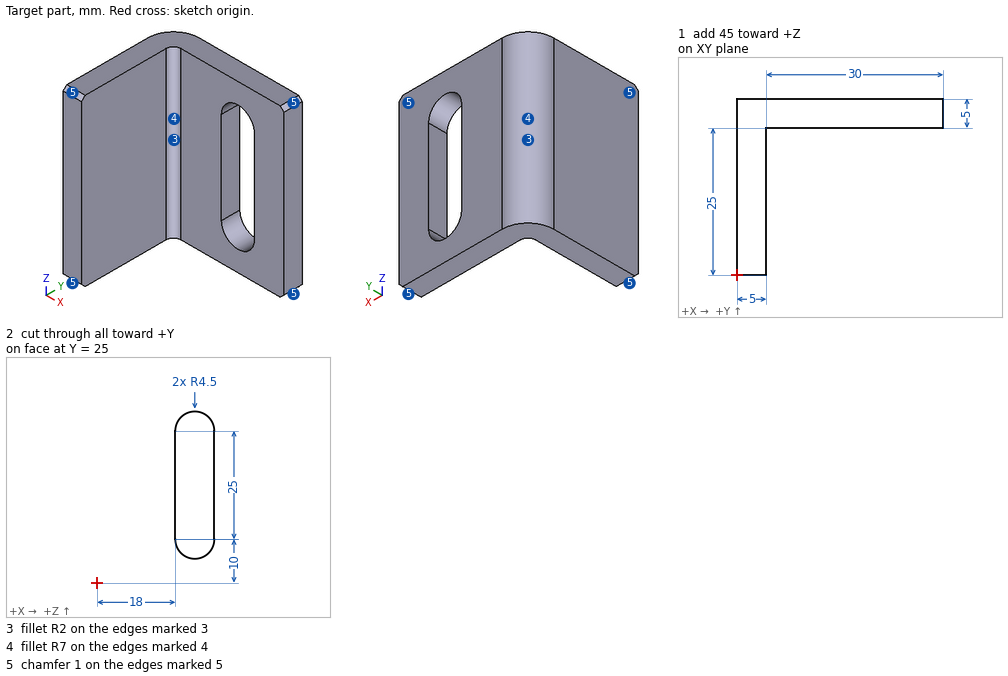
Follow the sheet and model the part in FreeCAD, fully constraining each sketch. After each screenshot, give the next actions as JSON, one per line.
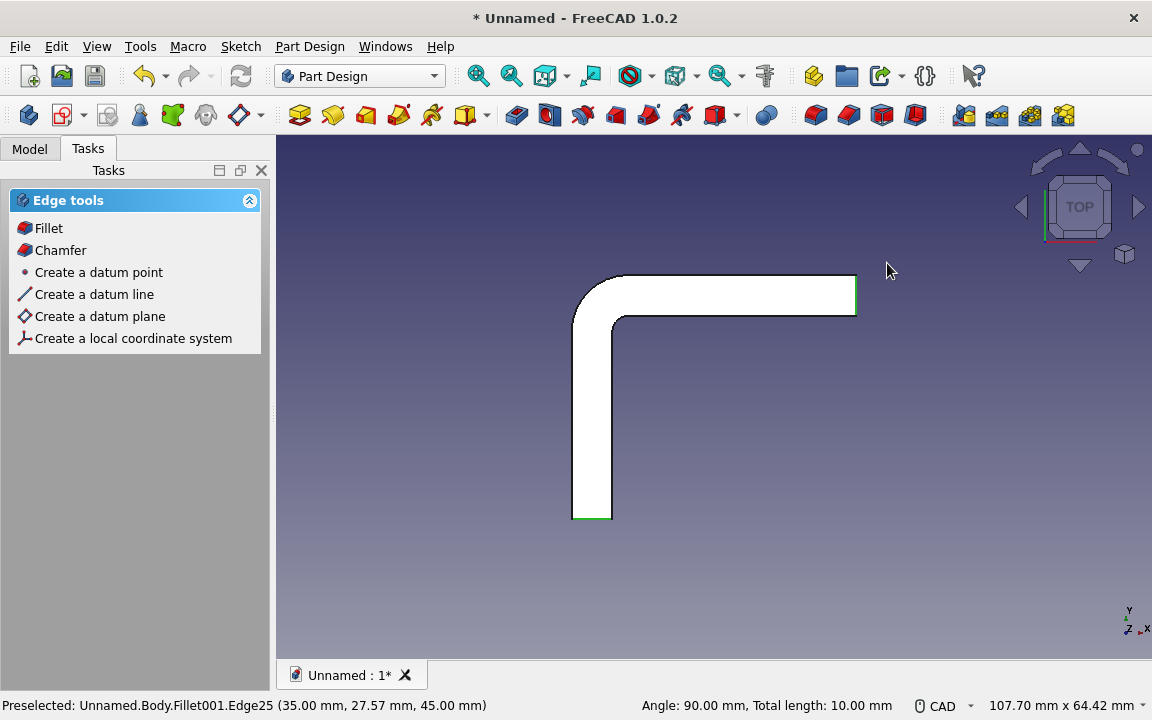
{"action": "key", "text": "1"}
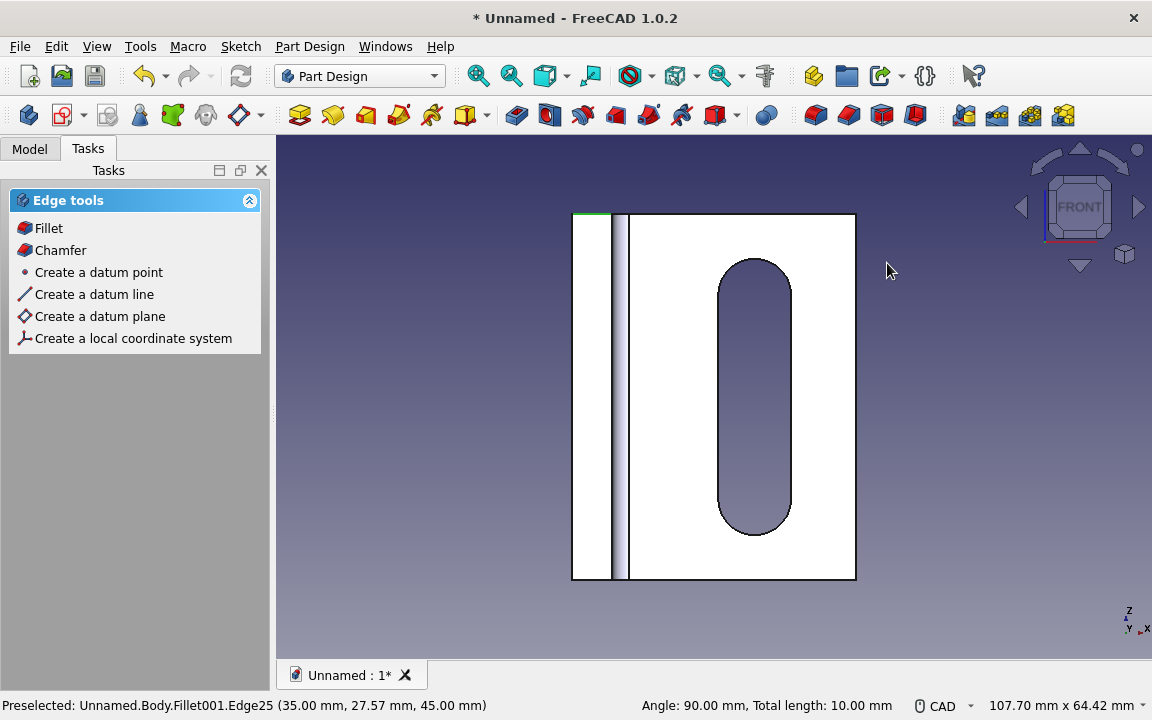
{"action": "left_click", "coordinate": [592, 579], "text": "ctrl"}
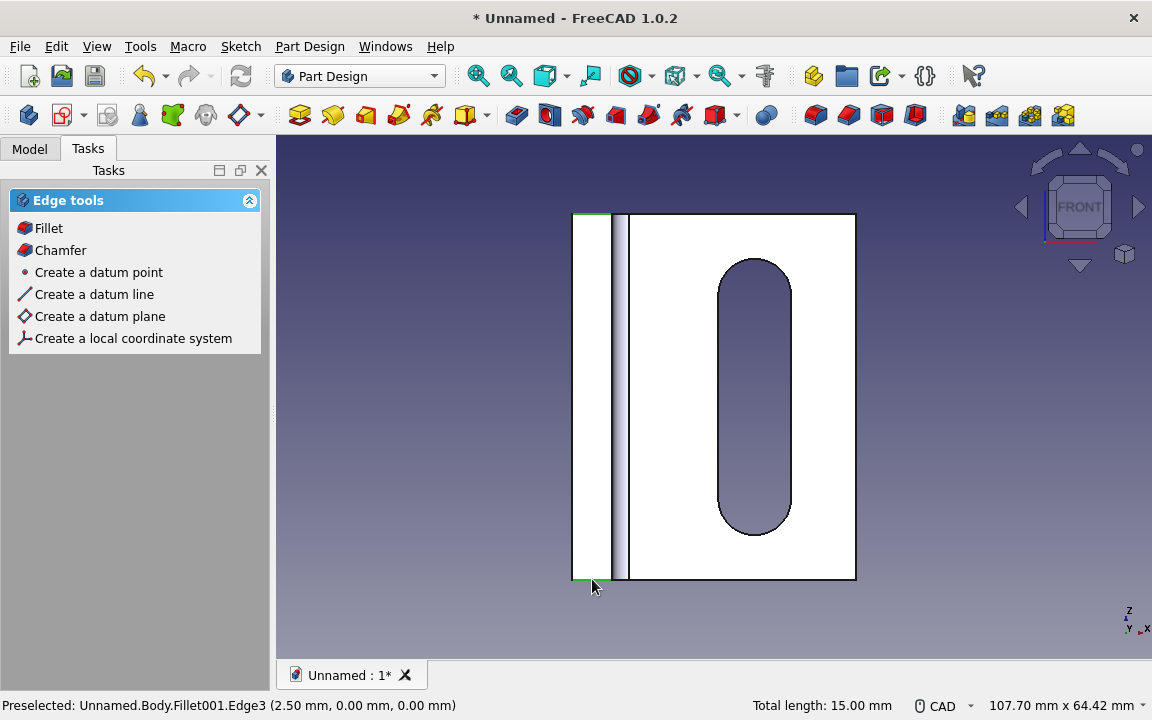
{"action": "key", "text": "3"}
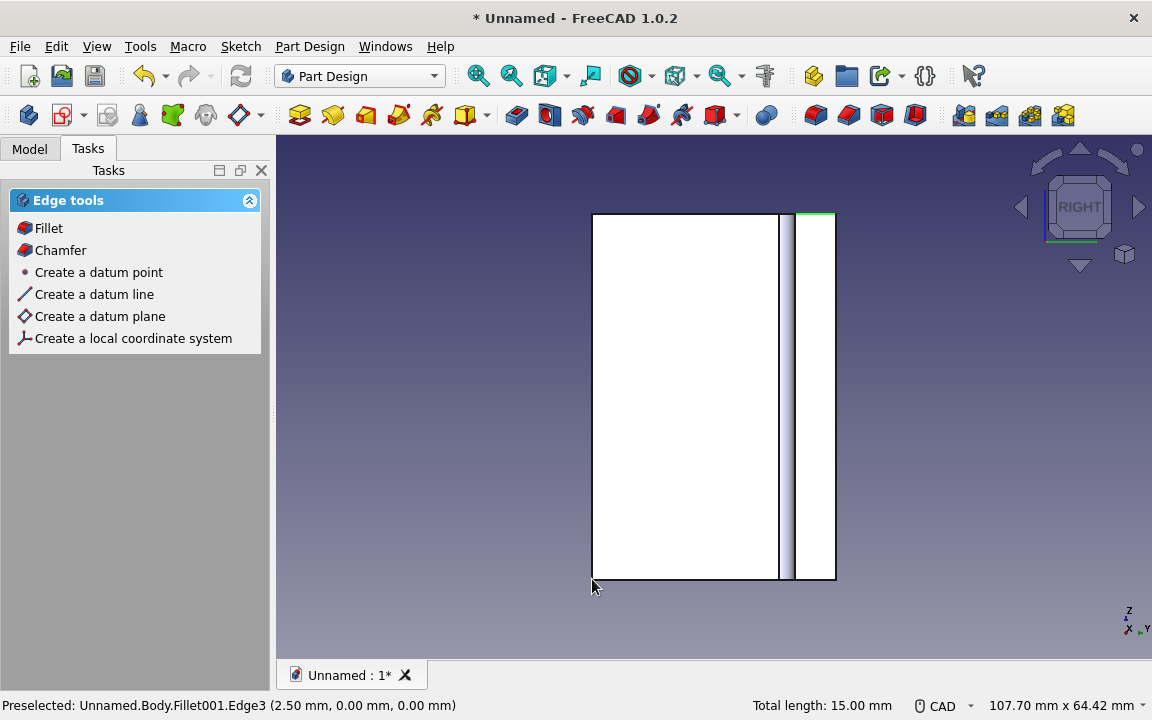
{"action": "left_click", "coordinate": [816, 579], "text": "ctrl"}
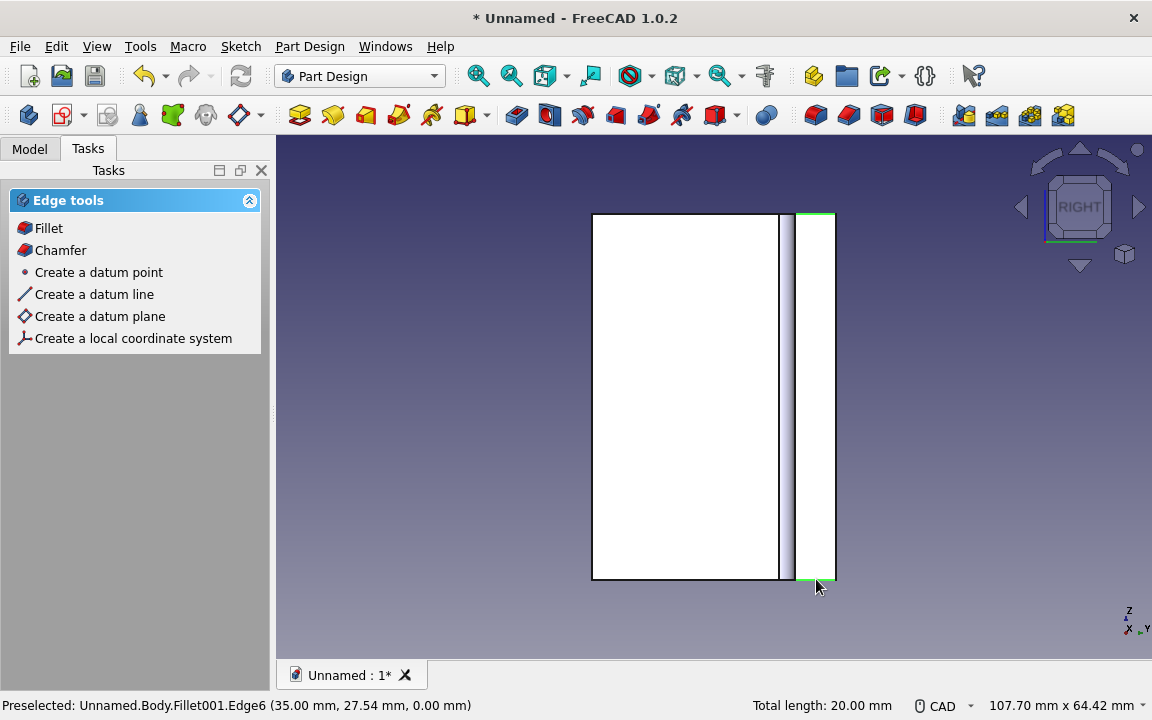
{"action": "left_click", "coordinate": [849, 116]}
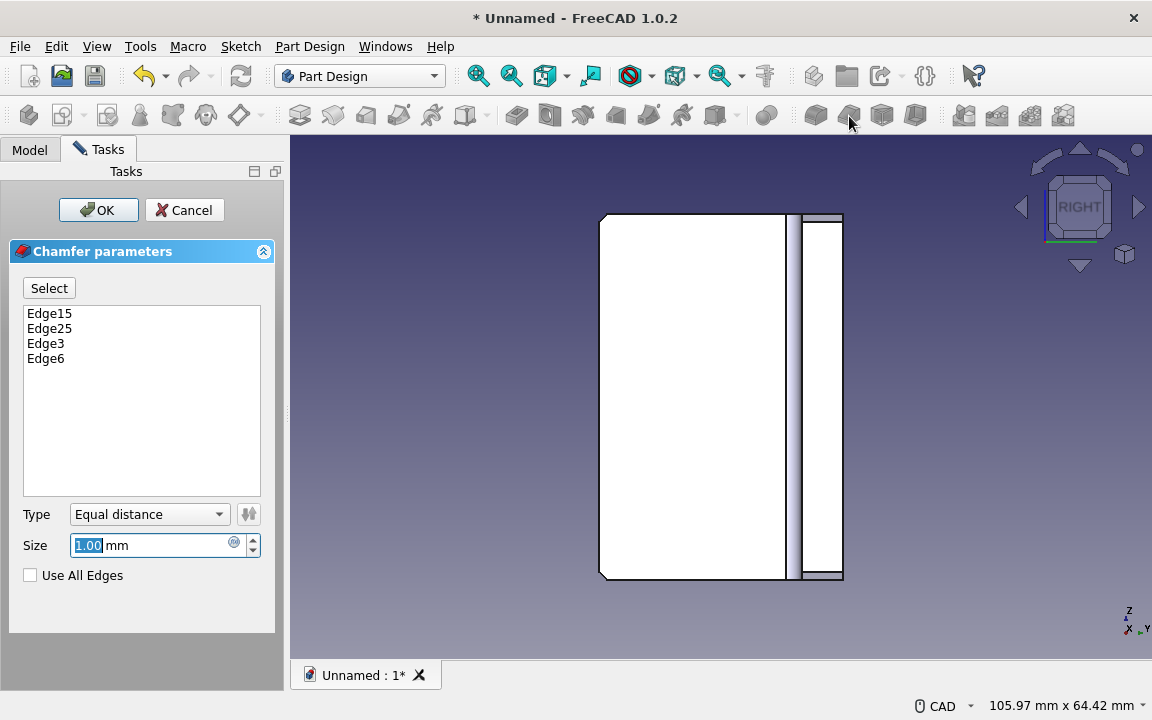
{"action": "type", "text": "1"}
{"action": "key", "text": "Tab"}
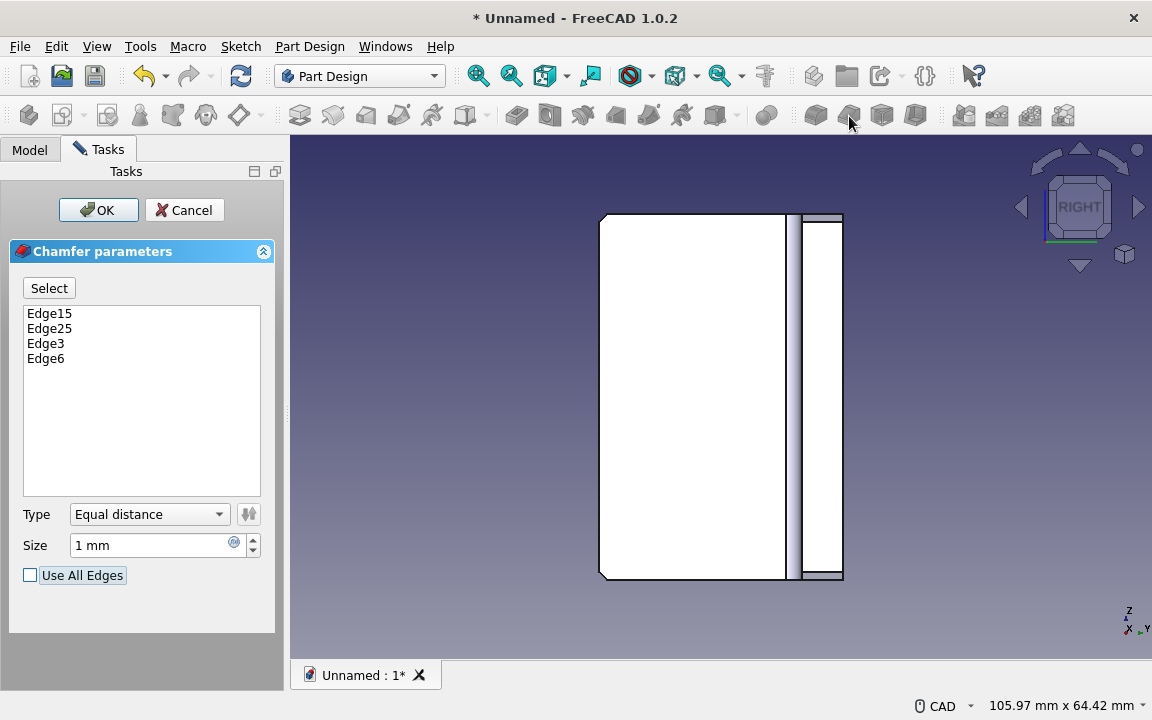
{"action": "left_click", "coordinate": [99, 210]}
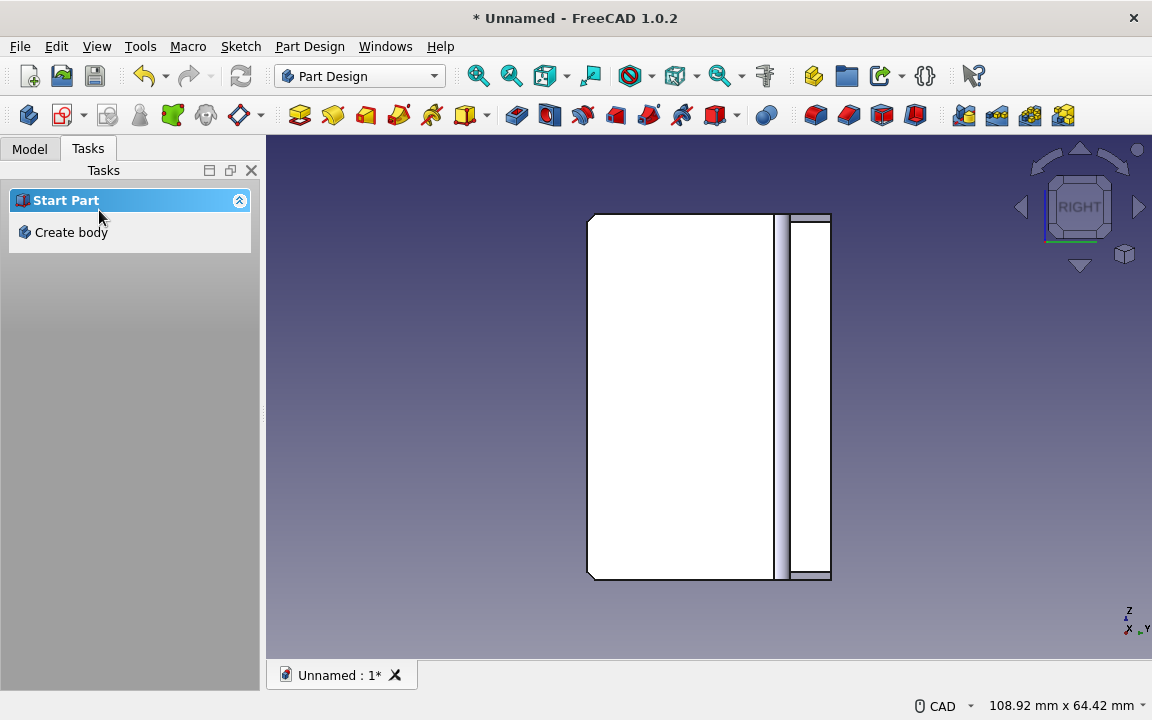
{"action": "key", "text": "0"}